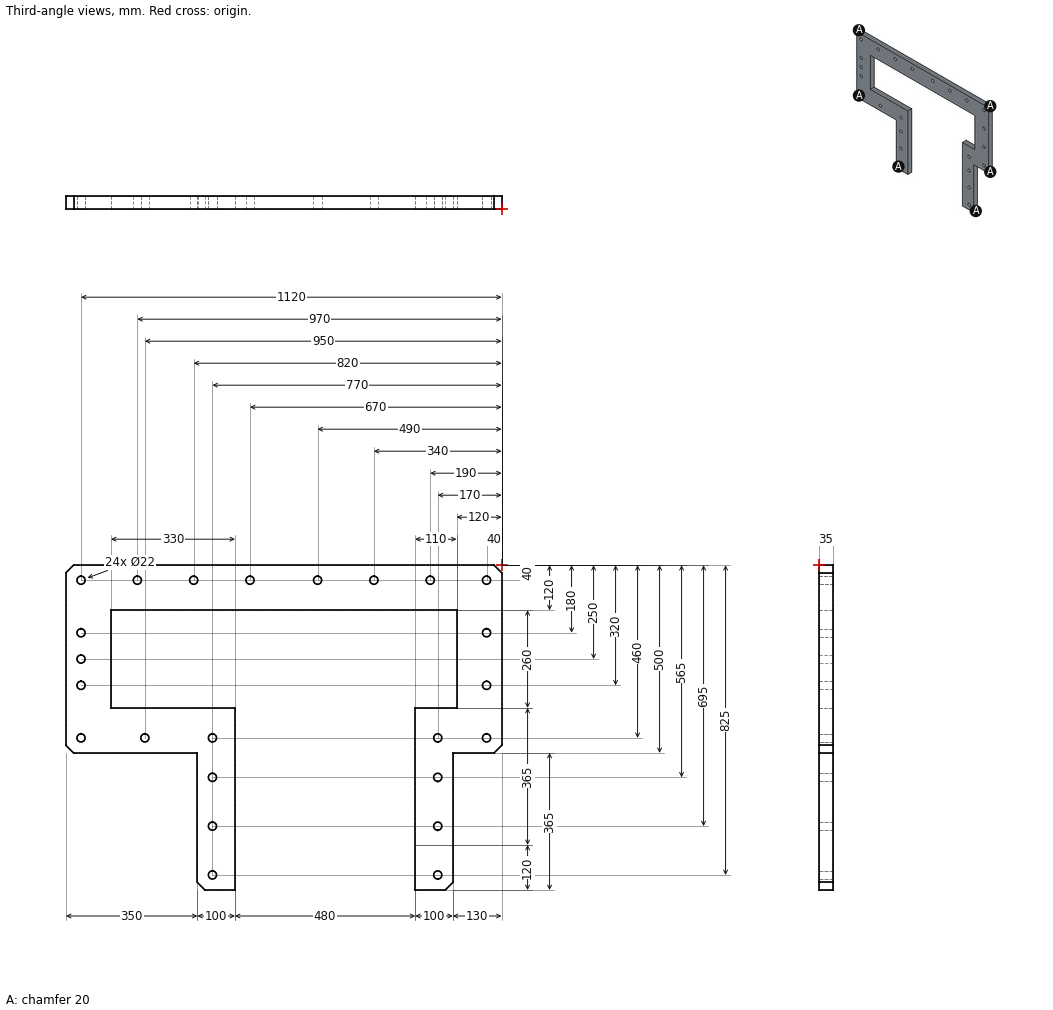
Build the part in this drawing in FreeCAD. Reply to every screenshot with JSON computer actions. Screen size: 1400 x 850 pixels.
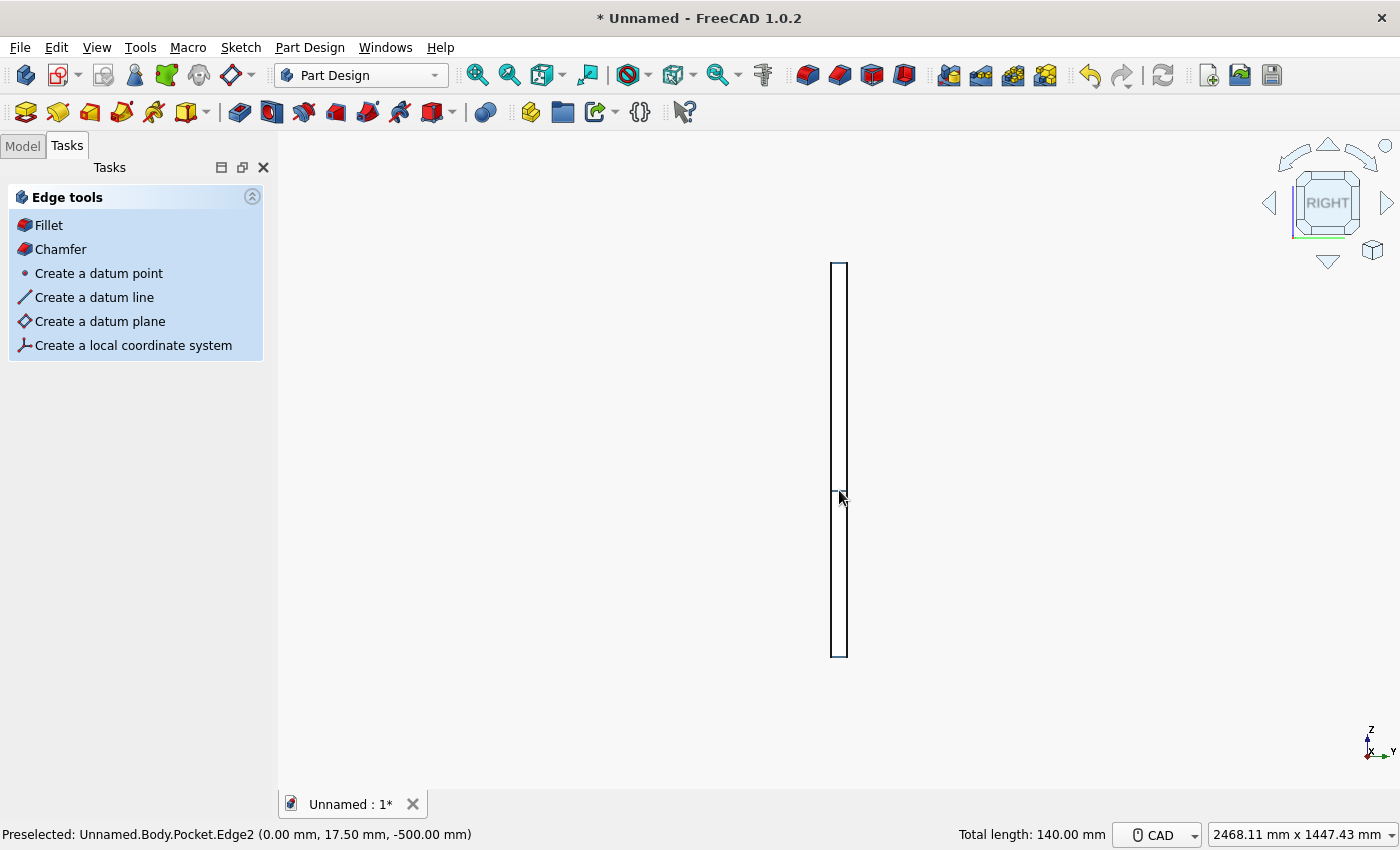
{"action": "scroll", "coordinate": [839, 490], "scroll_direction": "up", "scroll_amount": 5}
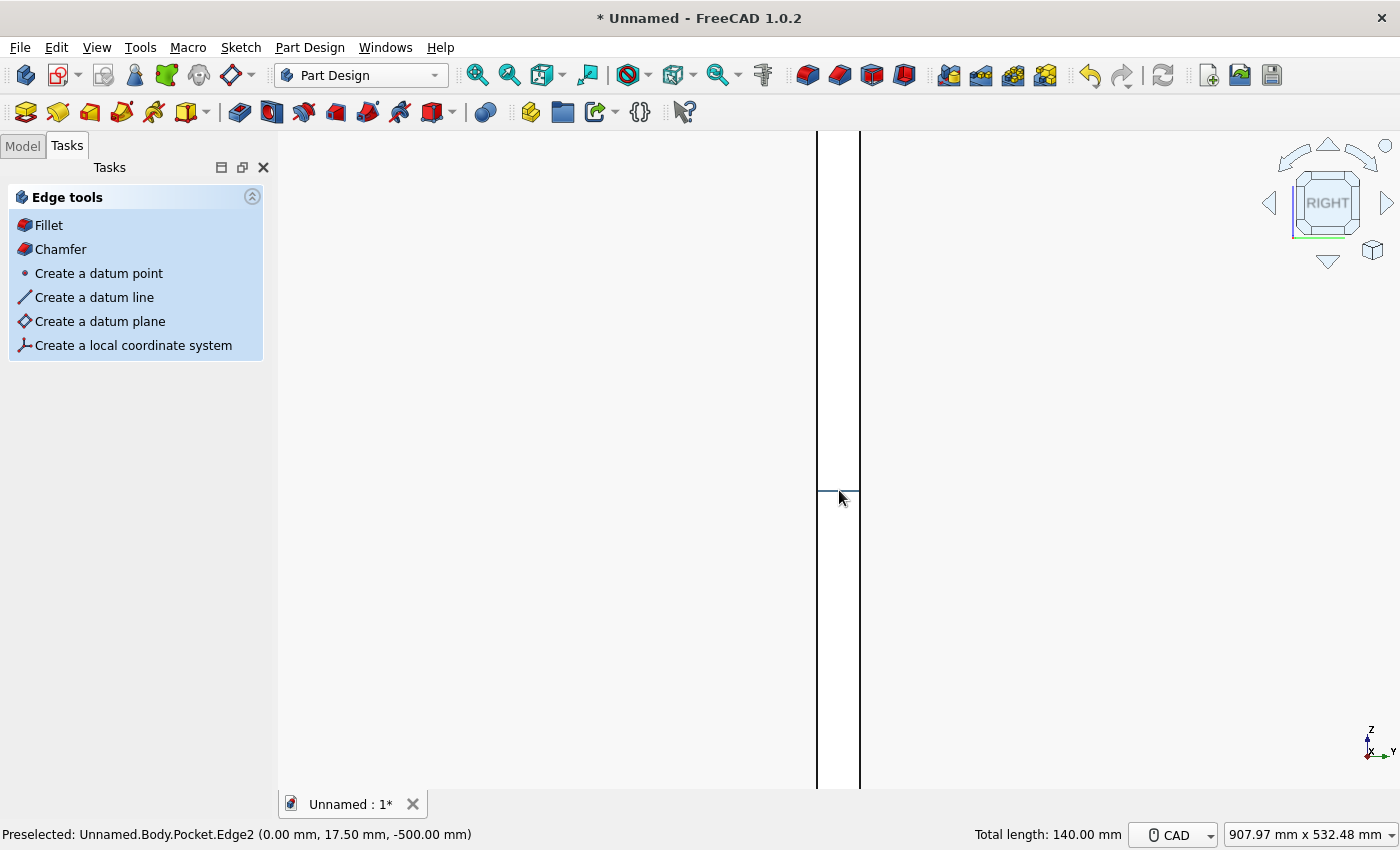
{"action": "key", "text": "v f"}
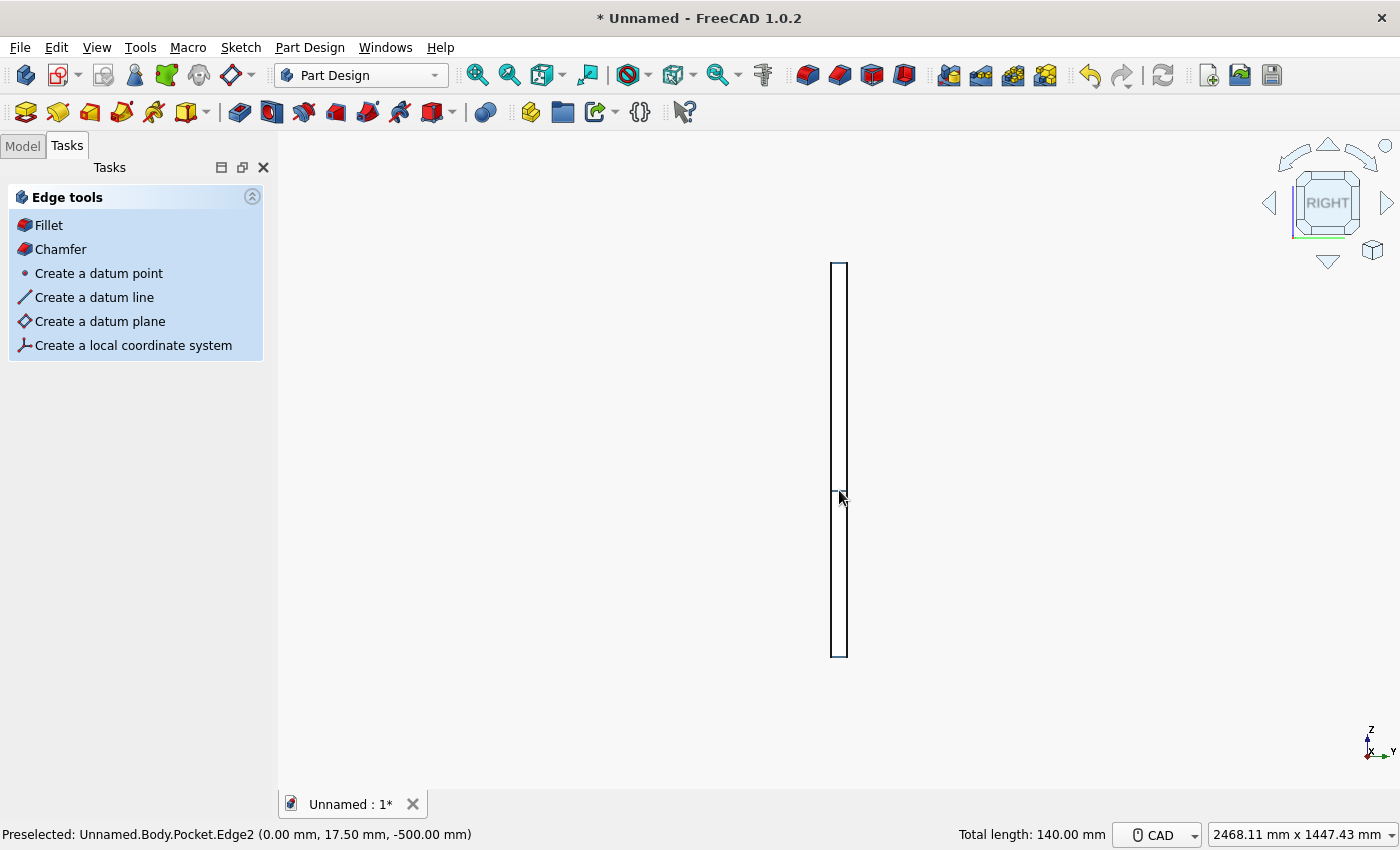
{"action": "key", "text": "5"}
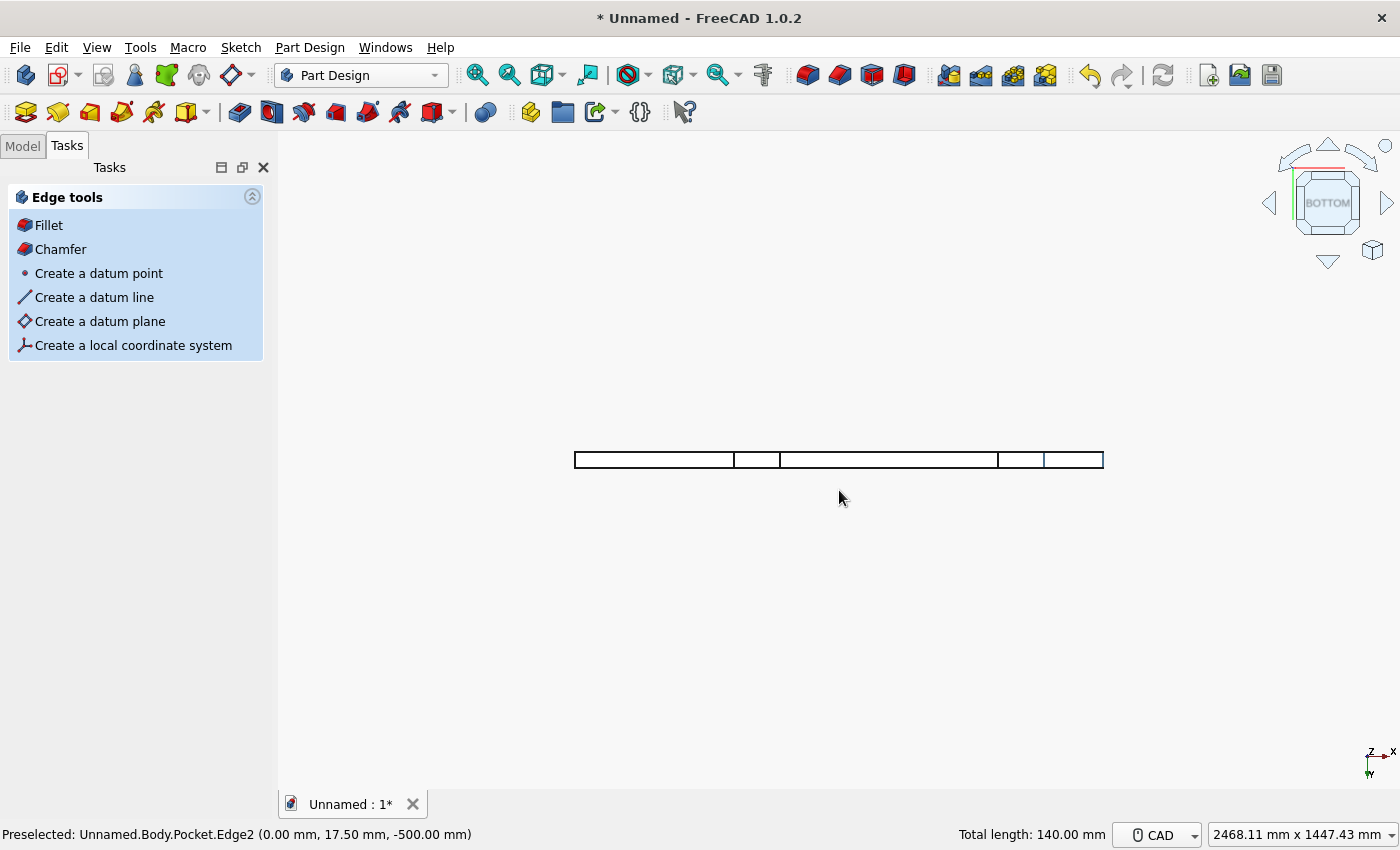
{"action": "left_click", "coordinate": [575, 459], "text": "ctrl"}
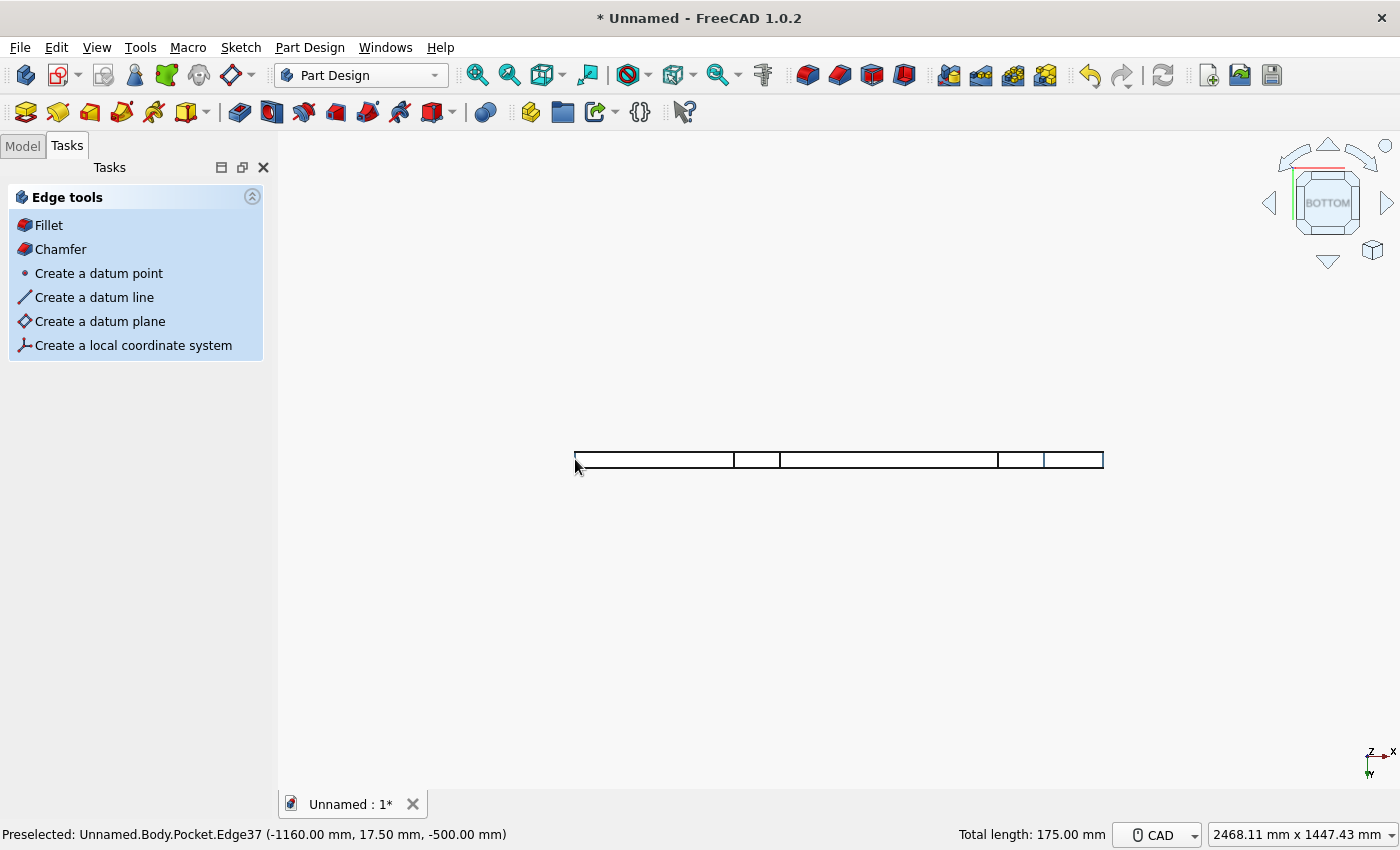
{"action": "left_click", "coordinate": [734, 459], "text": "ctrl"}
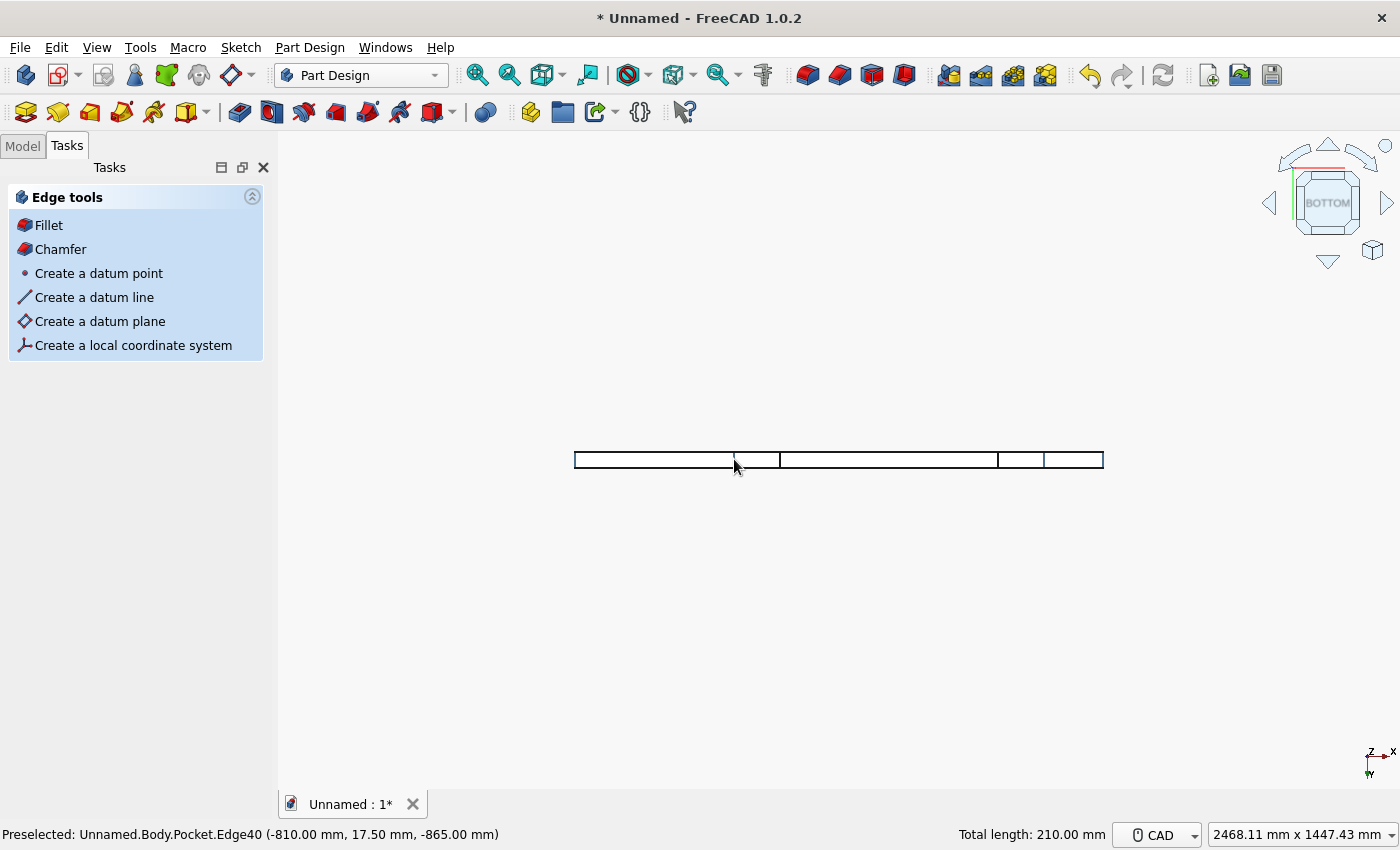
{"action": "left_click", "coordinate": [840, 76]}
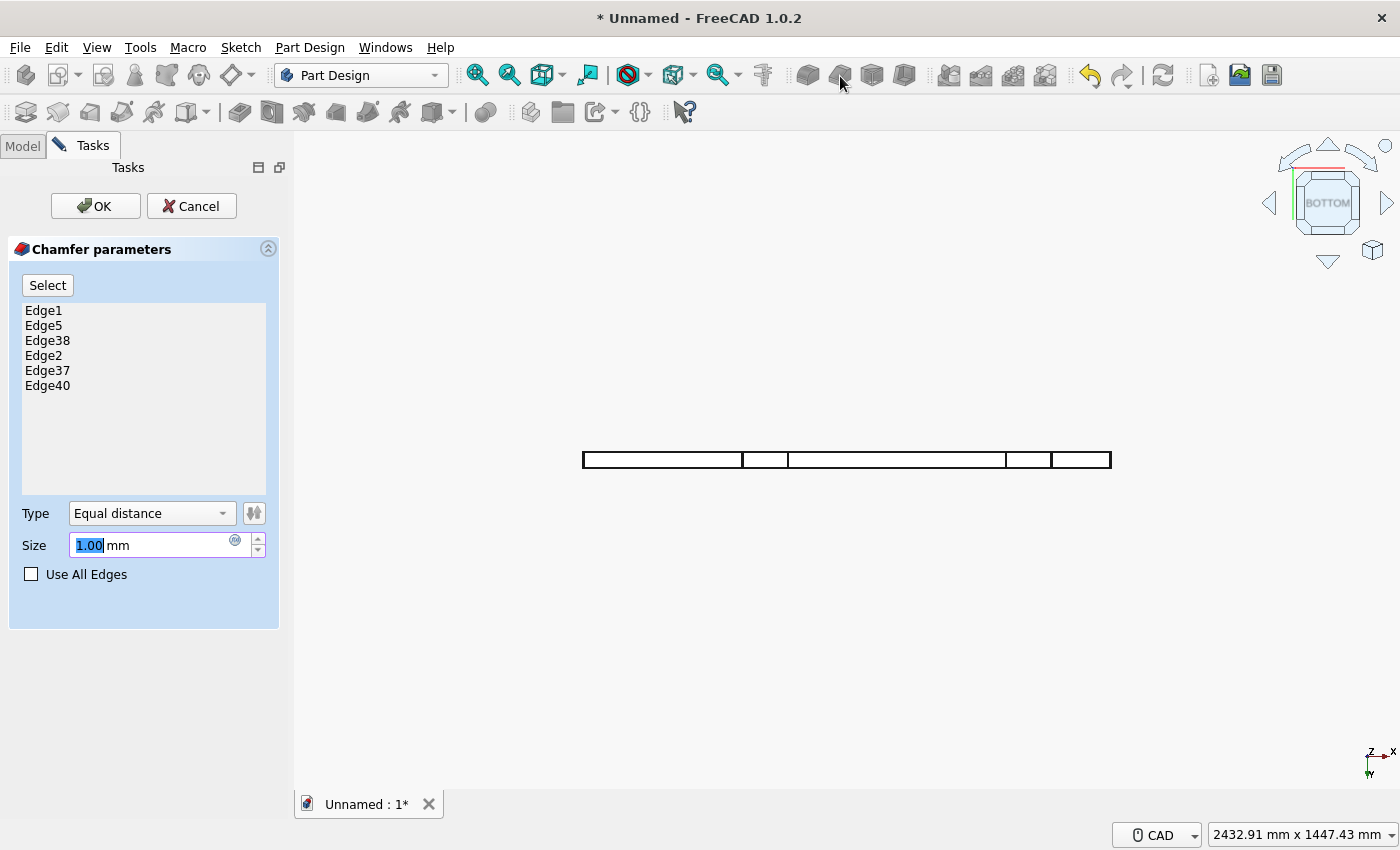
{"action": "type", "text": "20"}
{"action": "key", "text": "Tab"}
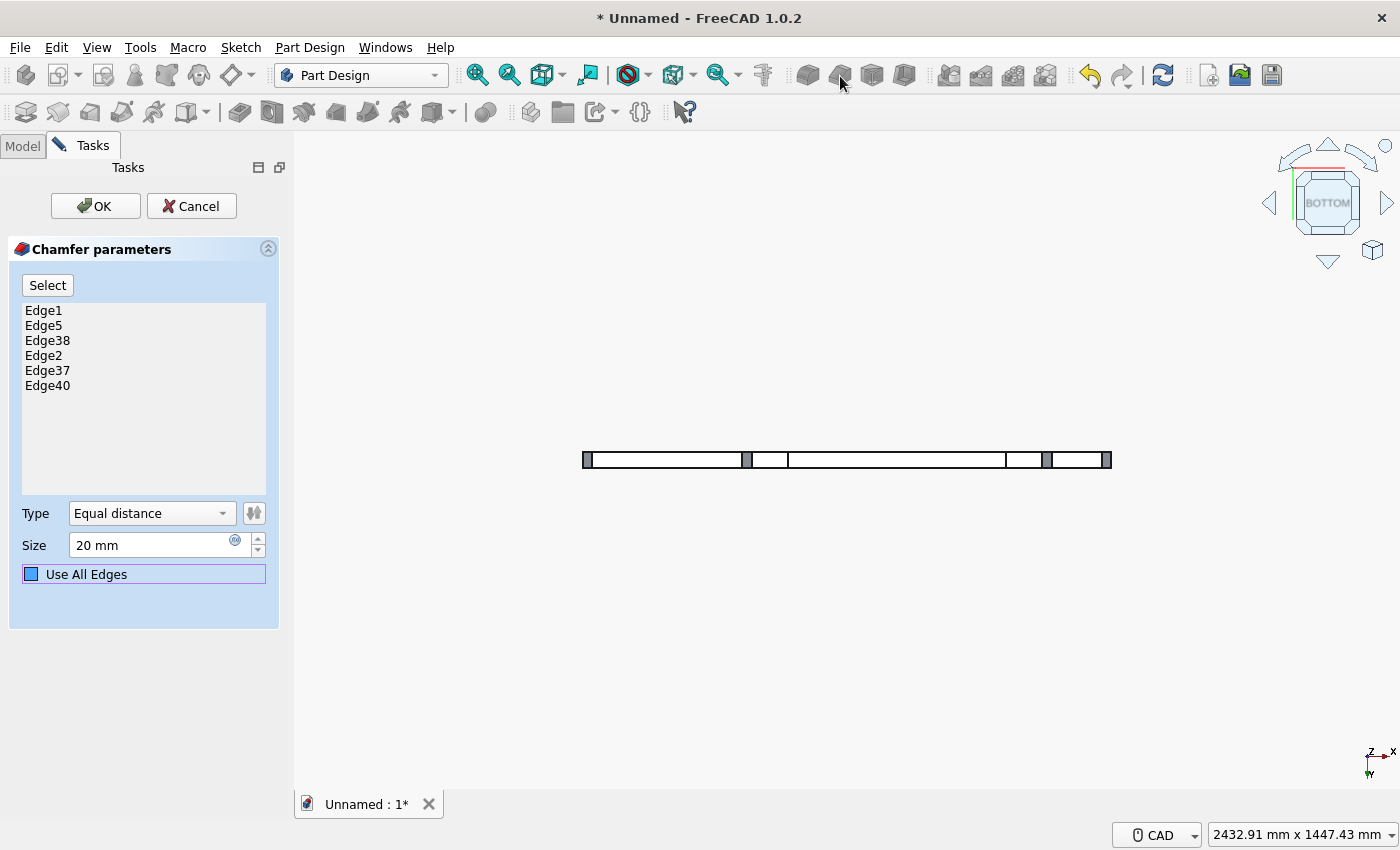
{"action": "left_click", "coordinate": [96, 206]}